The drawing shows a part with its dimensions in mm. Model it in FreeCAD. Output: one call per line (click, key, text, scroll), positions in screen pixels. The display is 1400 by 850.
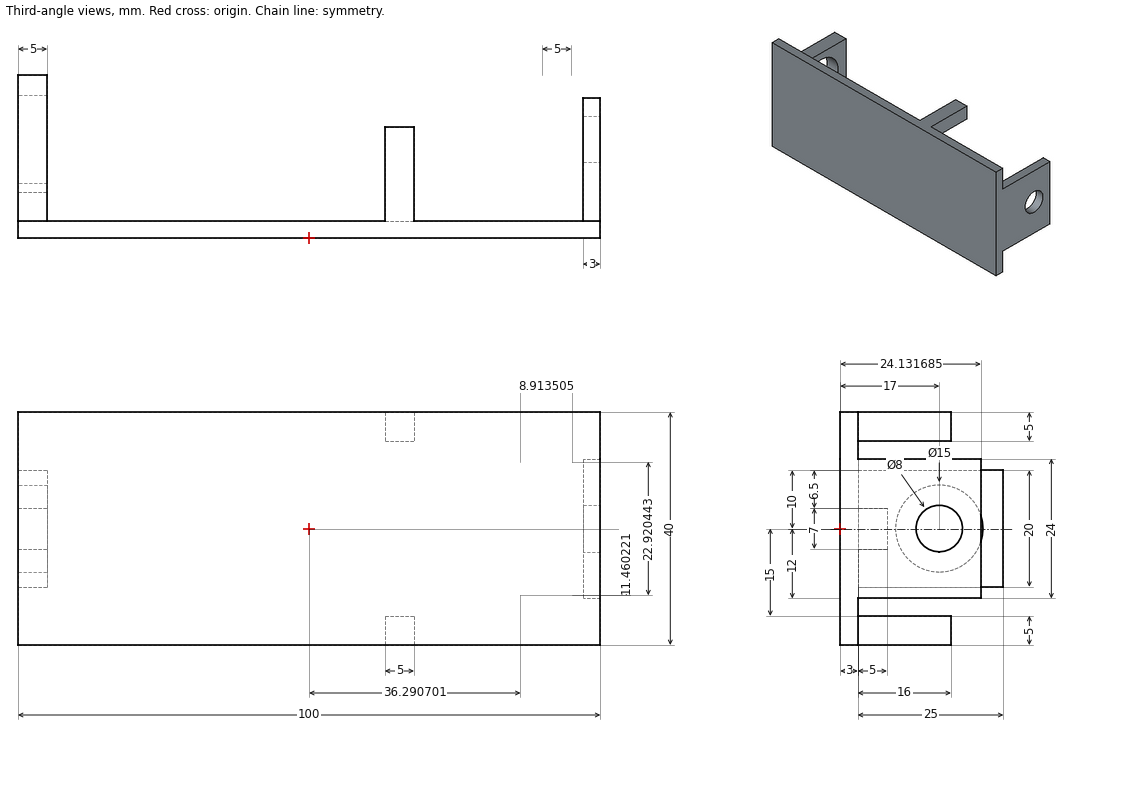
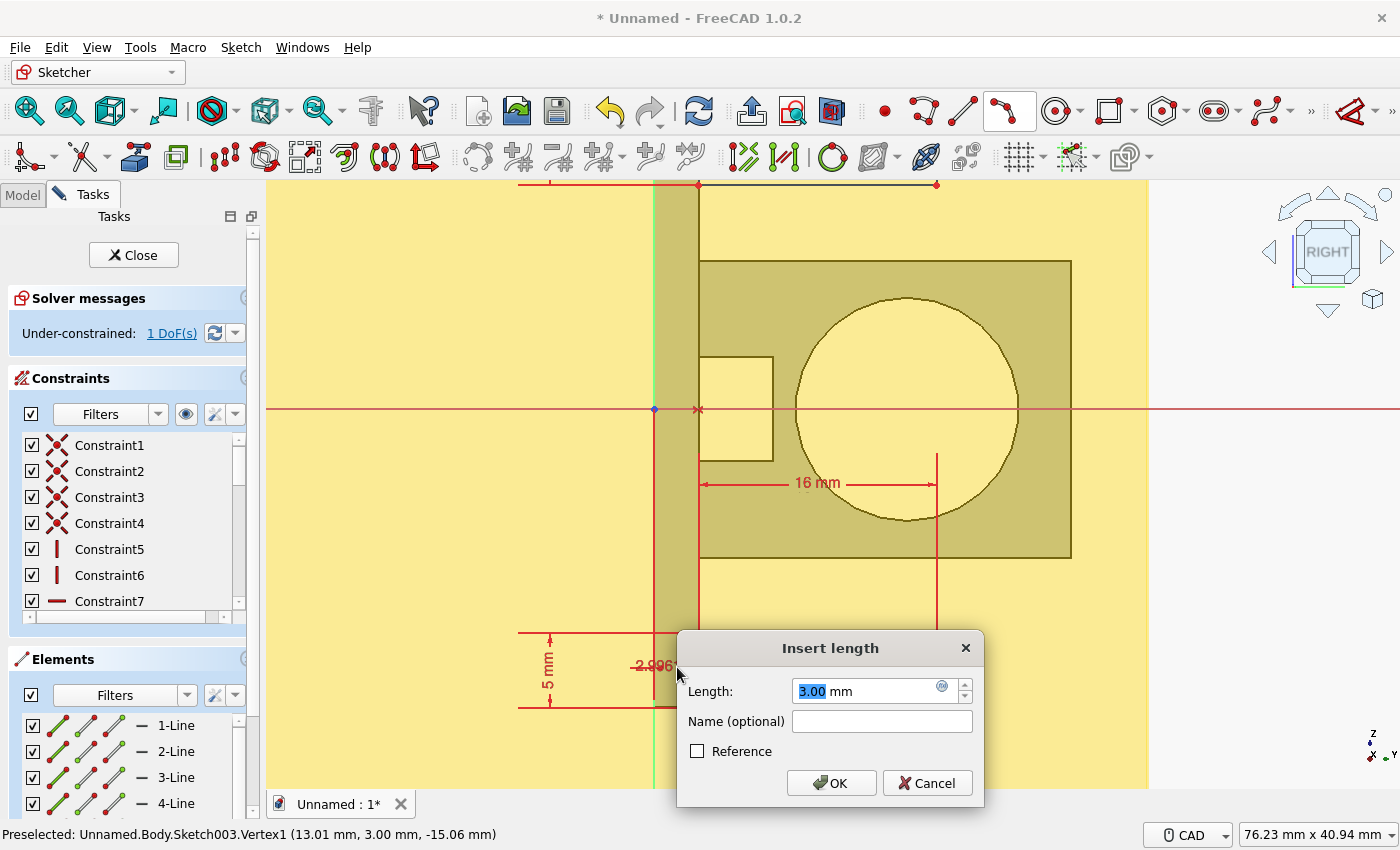
text(3)
key(Return)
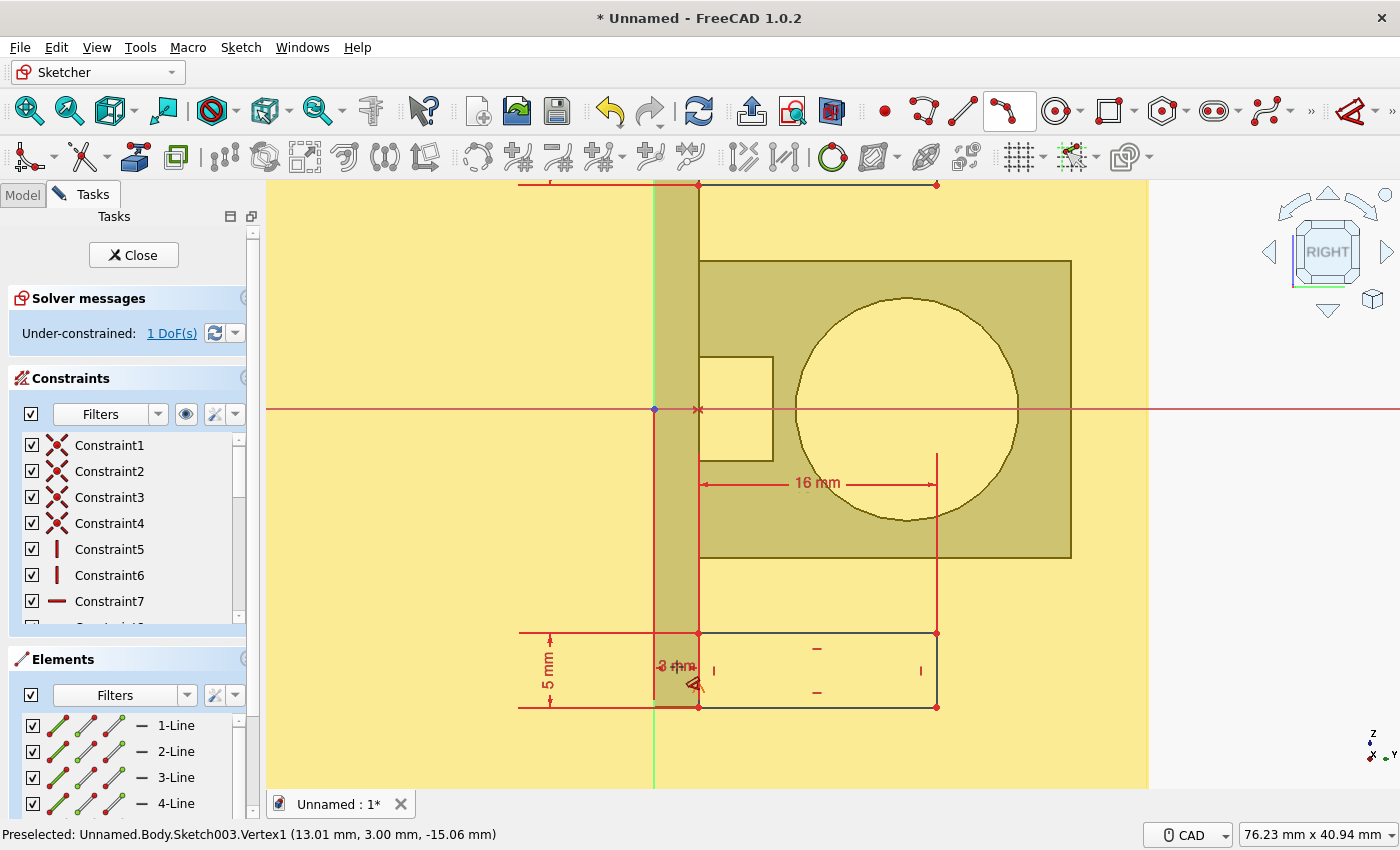
click(699, 633)
click(620, 521)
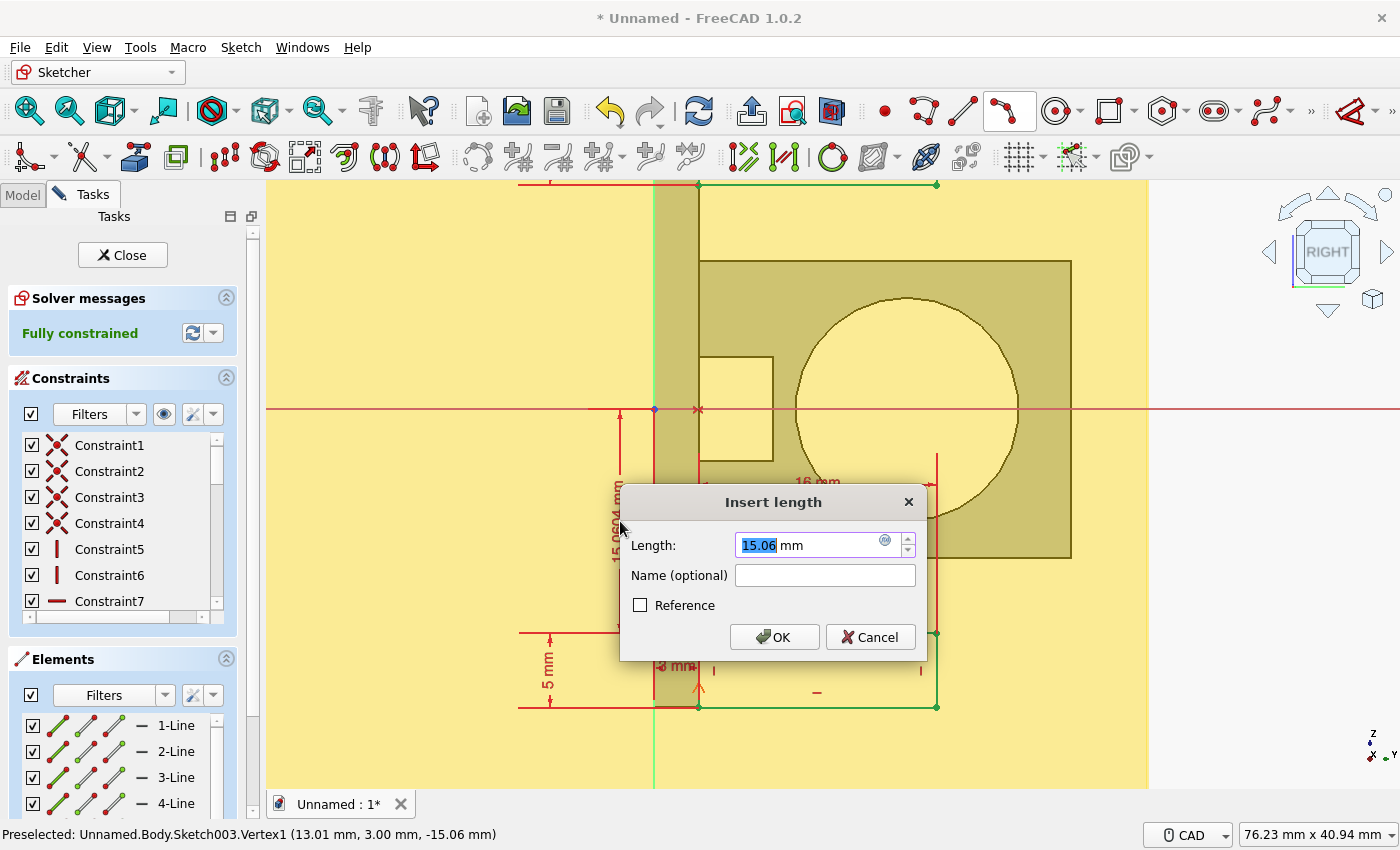
text(15)
key(Return)
key(Escape)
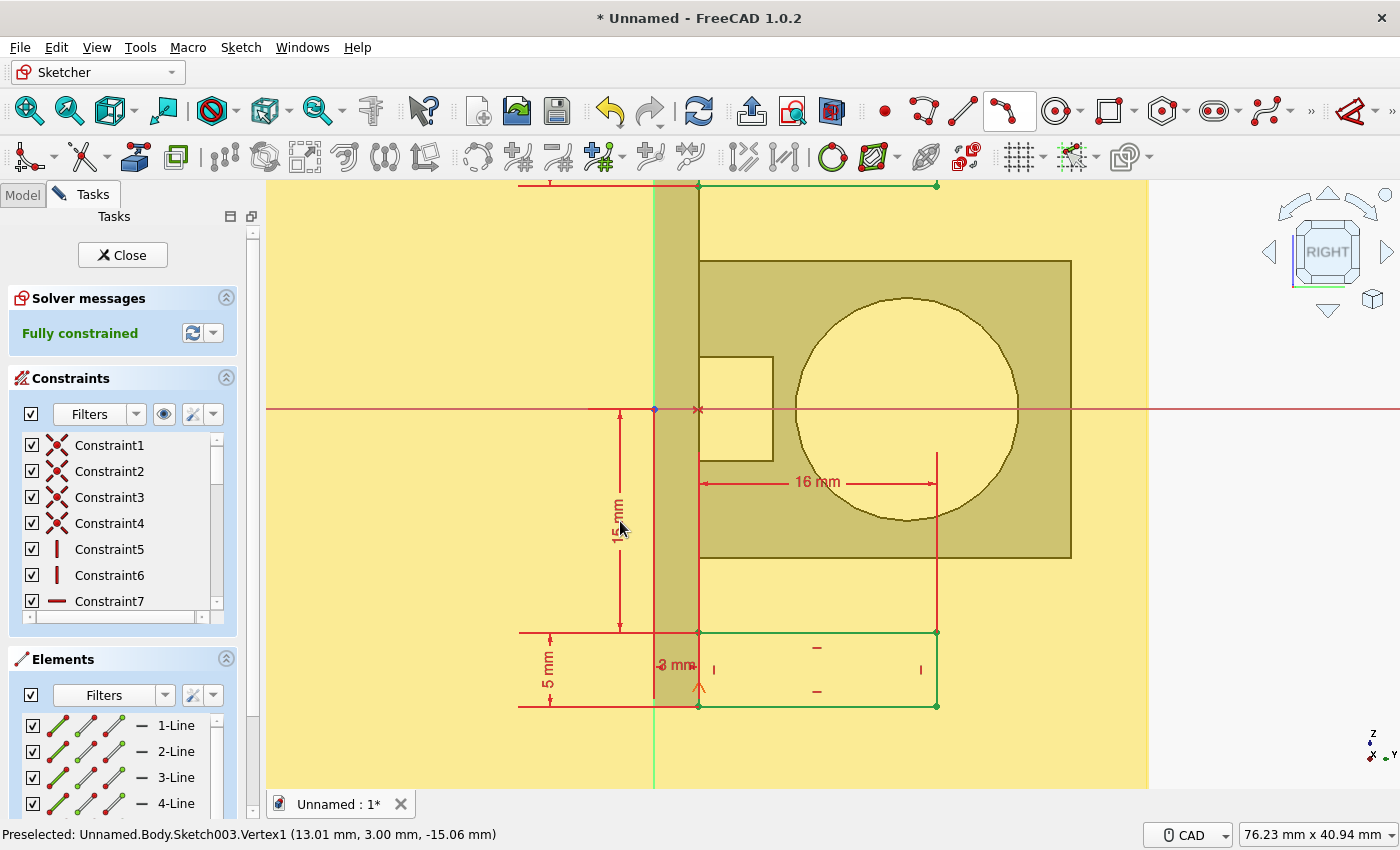
click(123, 255)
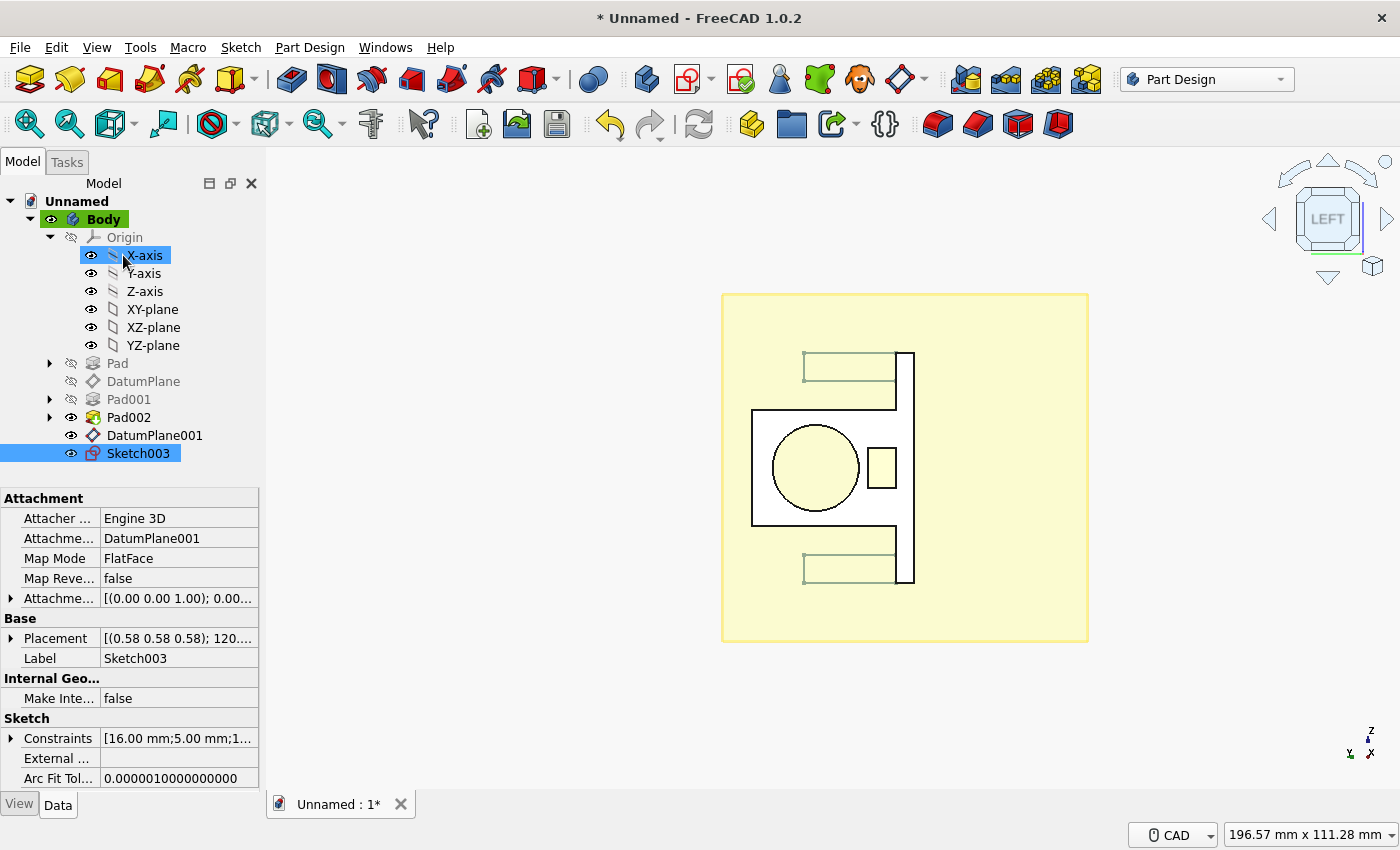
click(30, 80)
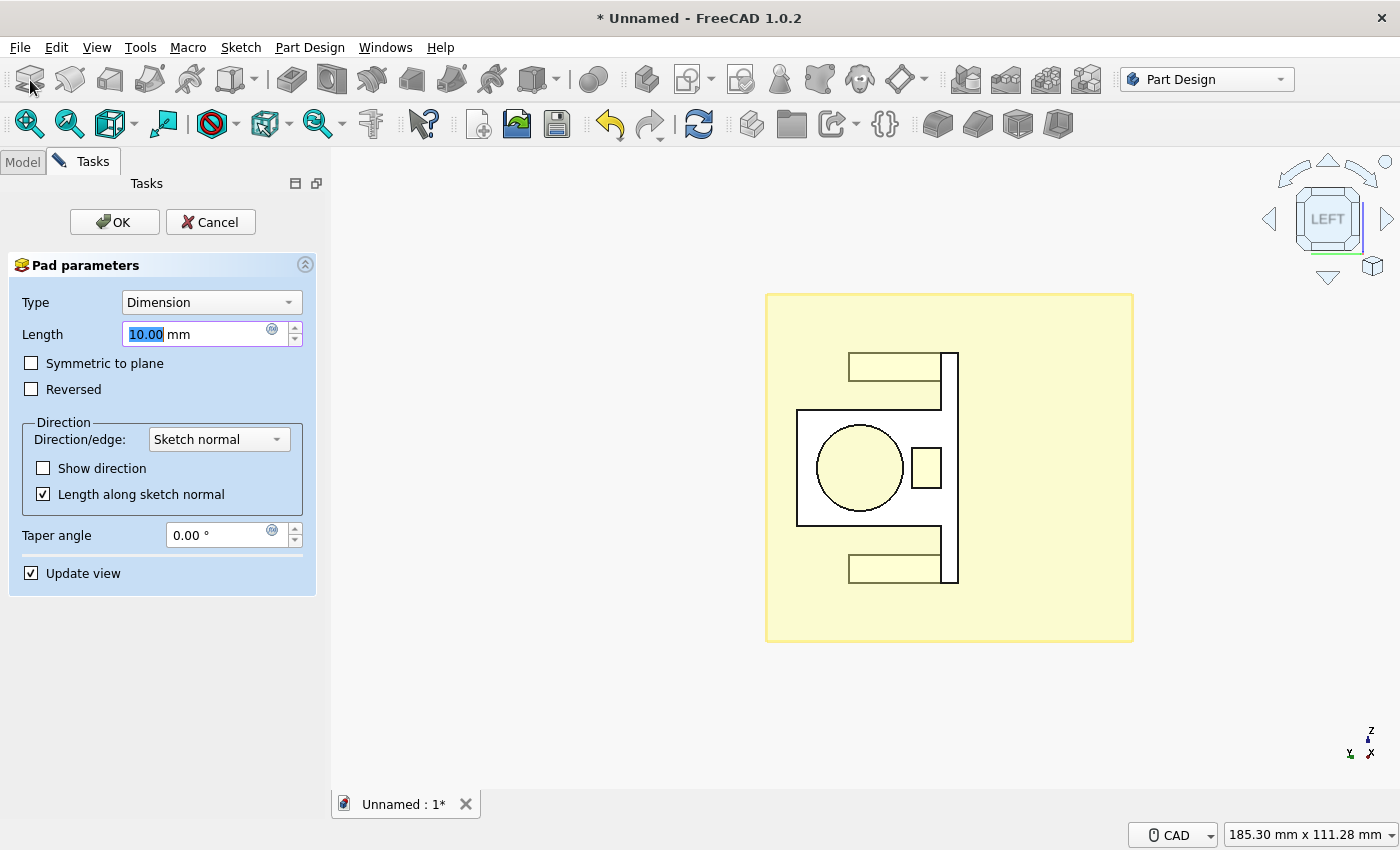
text(5)
key(Tab)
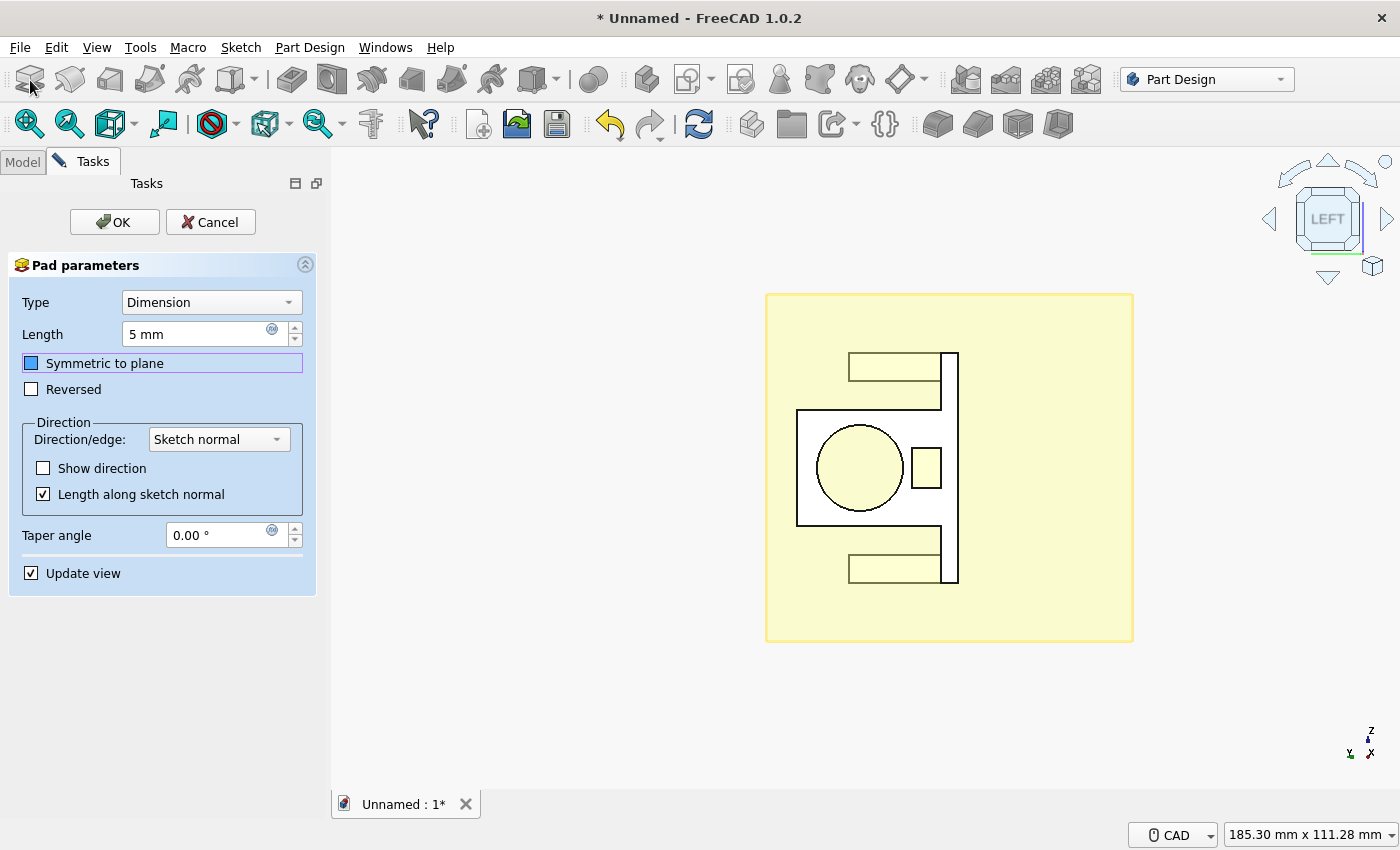
click(115, 222)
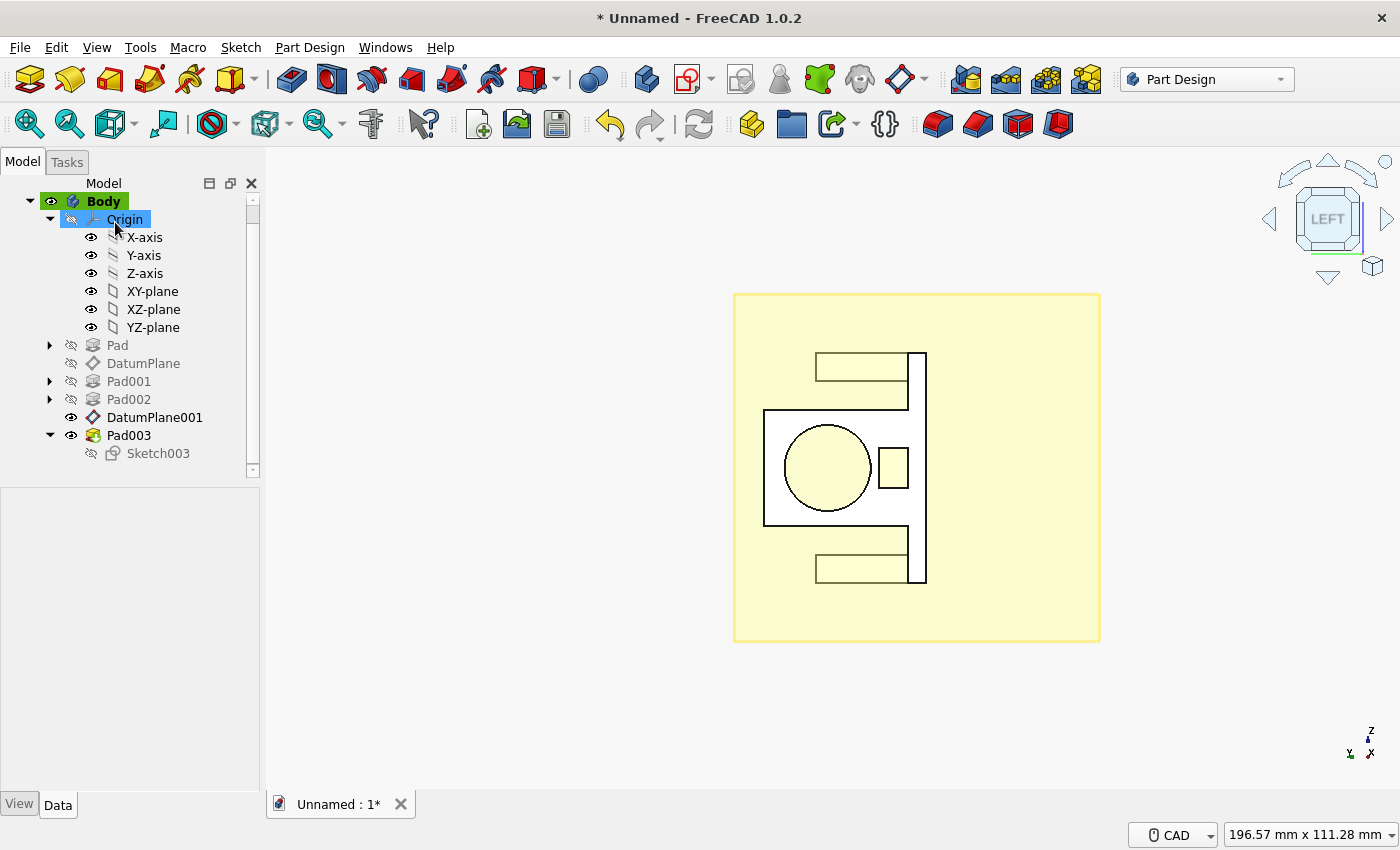
click(116, 417)
key(space)